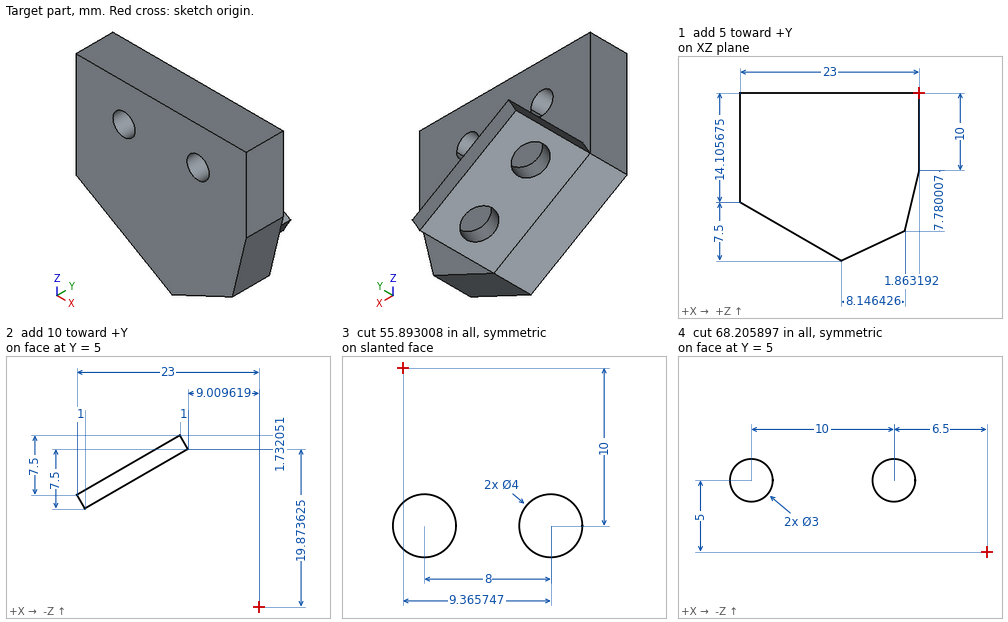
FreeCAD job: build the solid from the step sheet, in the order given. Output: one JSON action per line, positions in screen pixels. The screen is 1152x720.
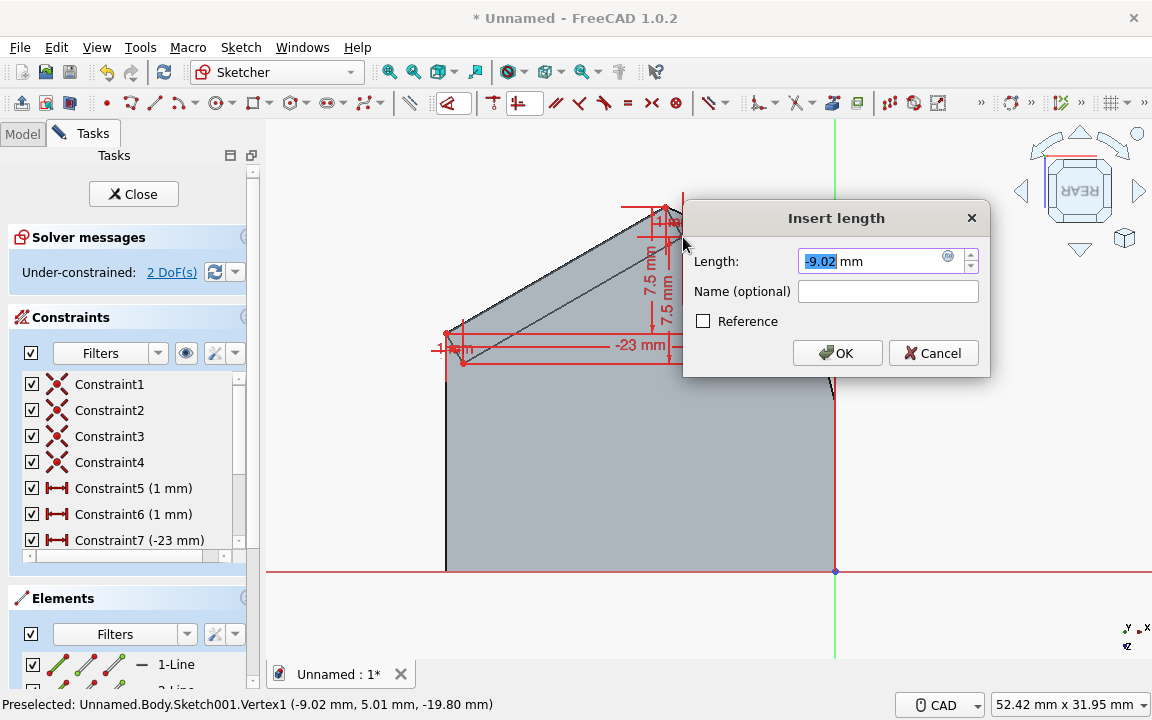
{"action": "type", "text": "-9.009619"}
{"action": "key", "text": "Return"}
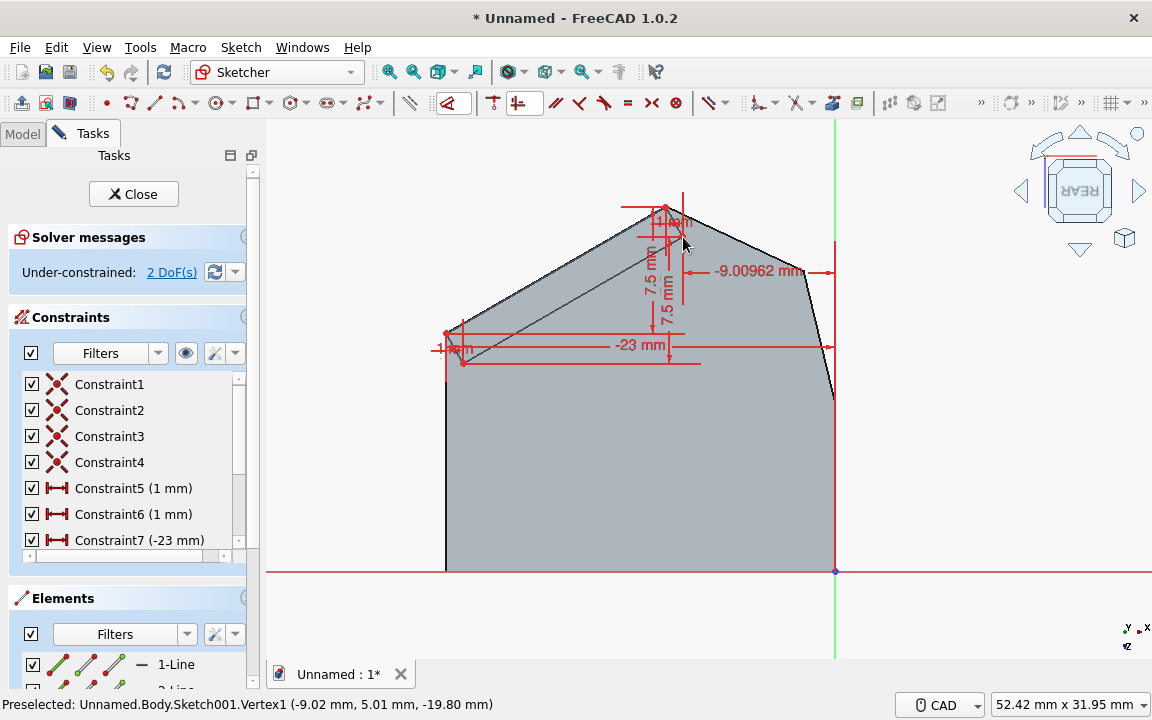
{"action": "scroll", "coordinate": [678, 228], "scroll_direction": "up", "scroll_amount": 2}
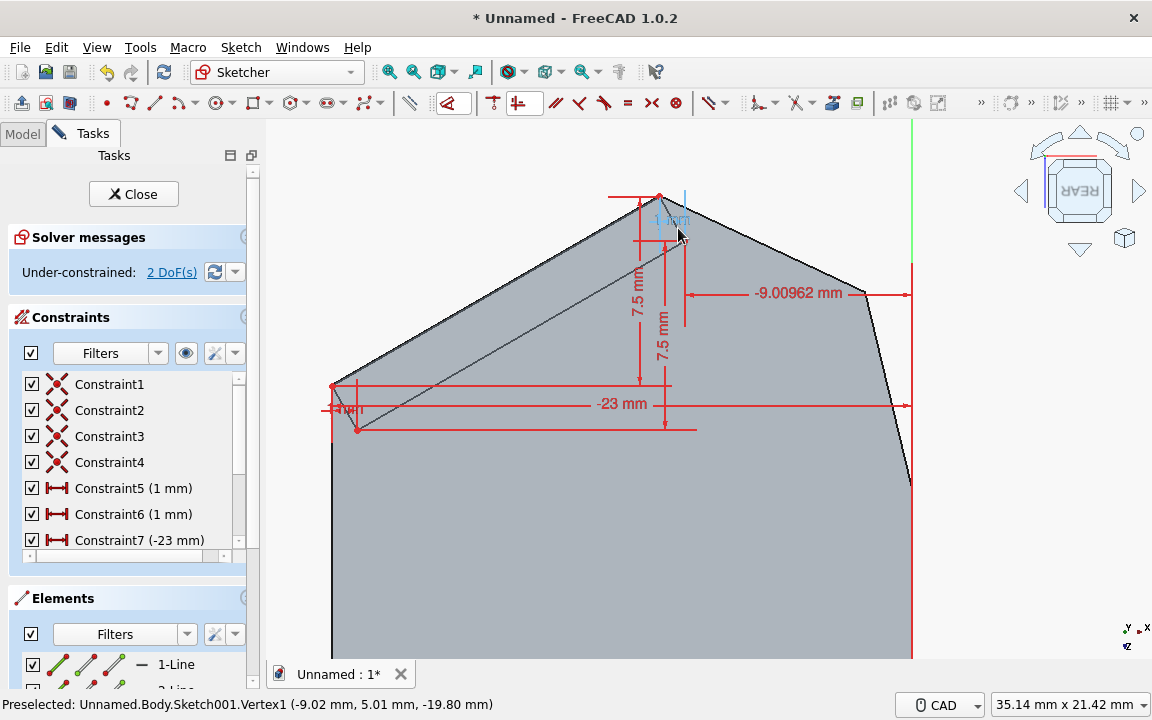
{"action": "left_click", "coordinate": [667, 210]}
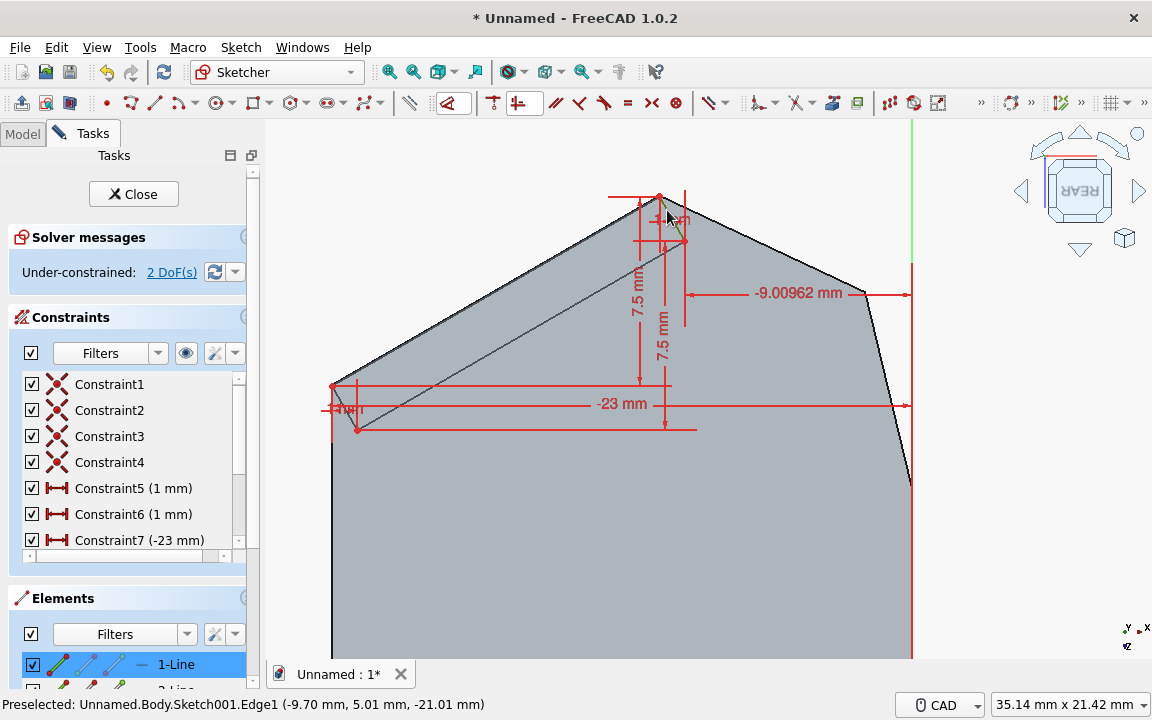
{"action": "key", "text": "i"}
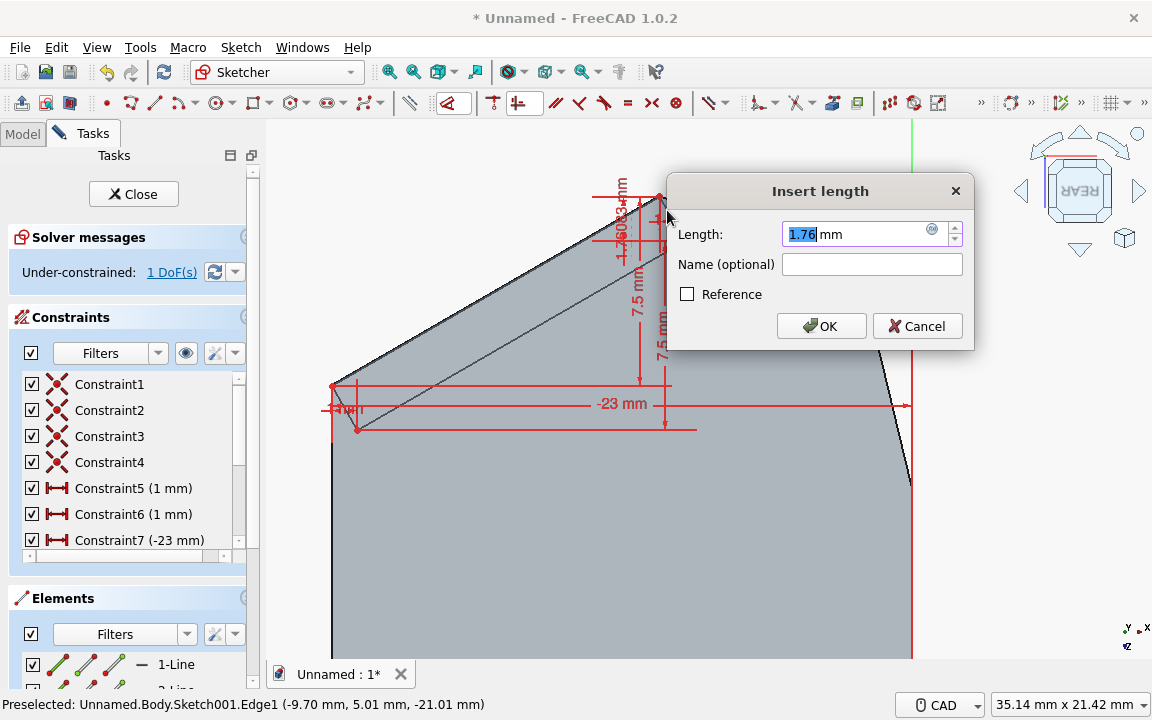
{"action": "type", "text": "1.732051"}
{"action": "key", "text": "Return"}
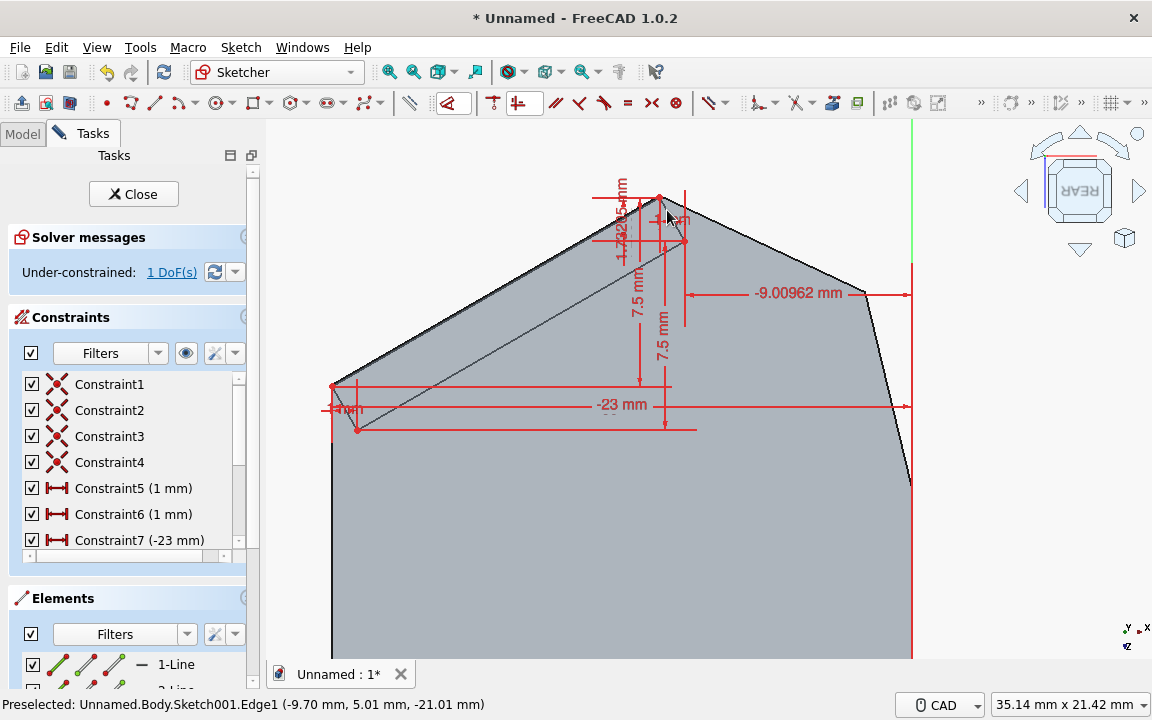
{"action": "left_click", "coordinate": [685, 241]}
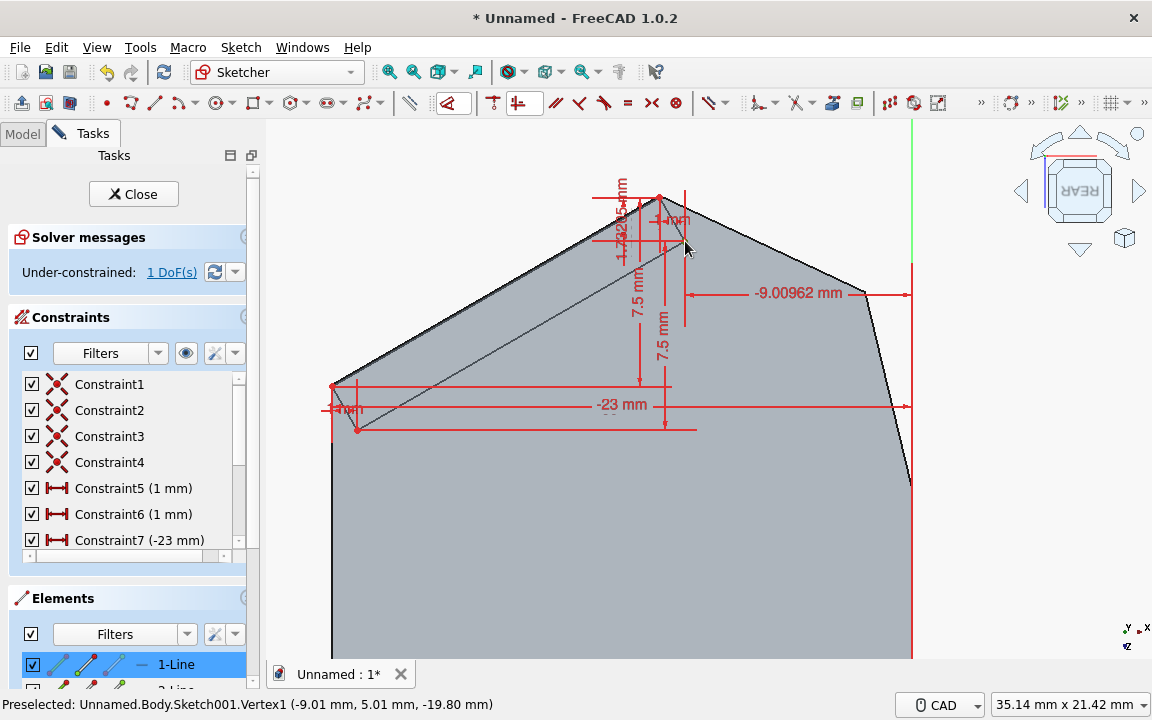
{"action": "key", "text": "i"}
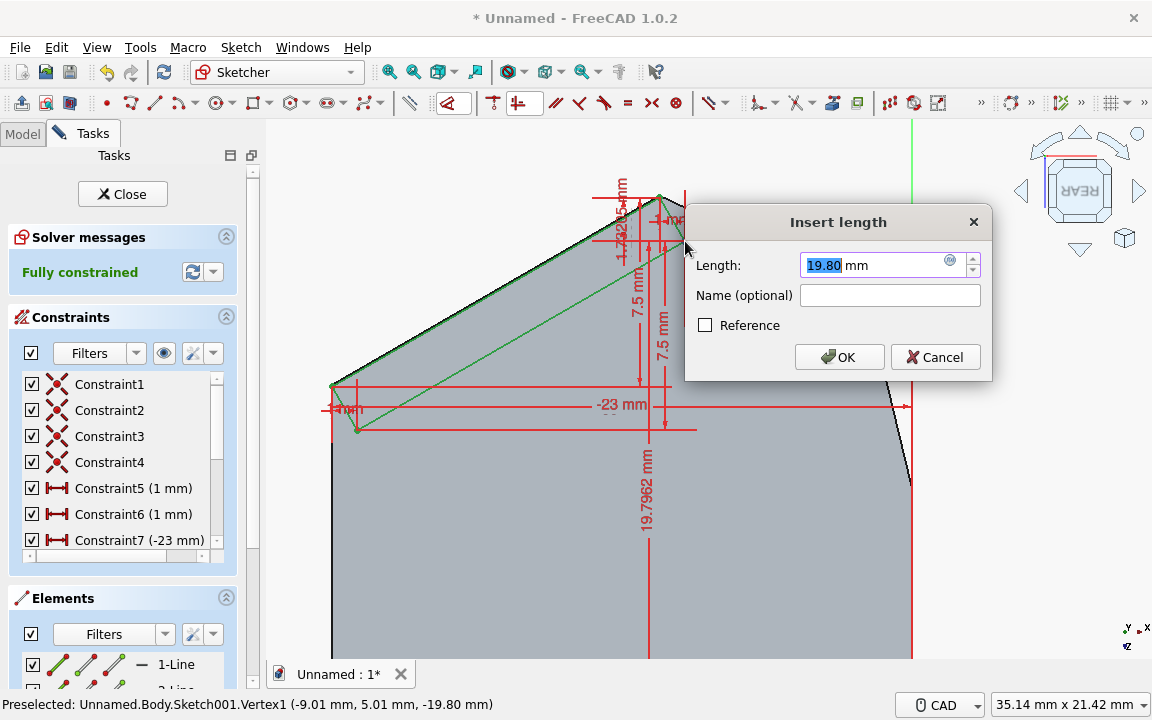
{"action": "type", "text": "19.873625"}
{"action": "key", "text": "Return"}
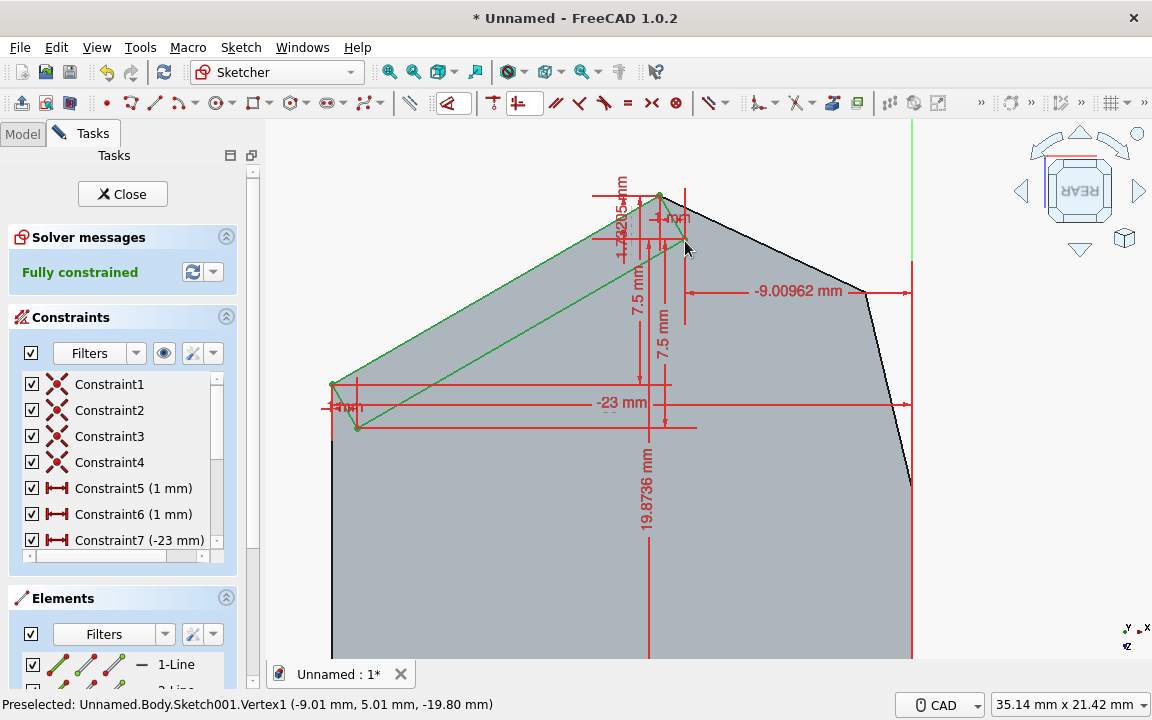
{"action": "left_click", "coordinate": [123, 194]}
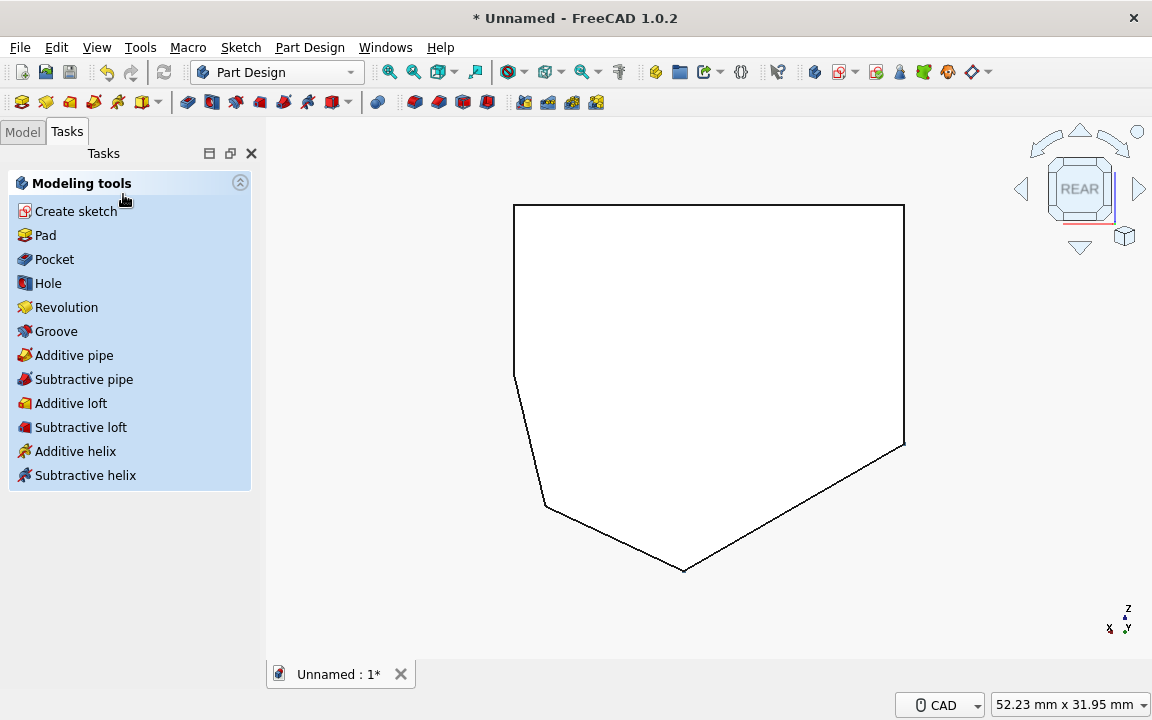
{"action": "left_click", "coordinate": [22, 102]}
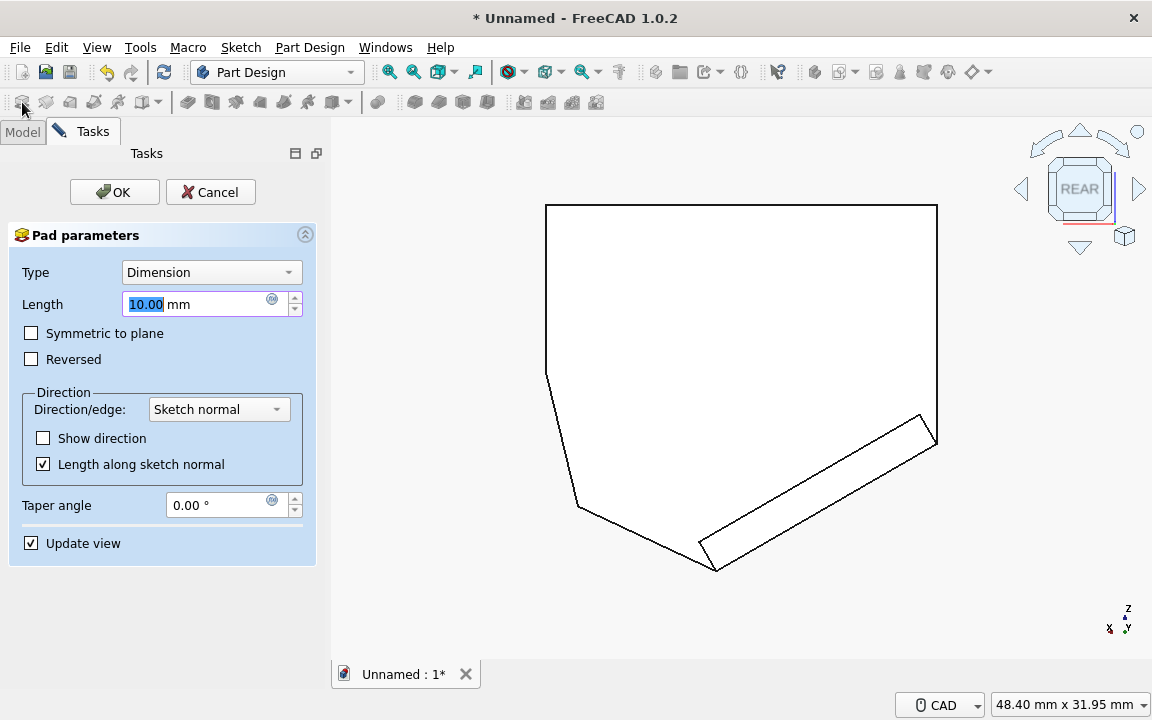
{"action": "type", "text": "10"}
{"action": "key", "text": "Tab"}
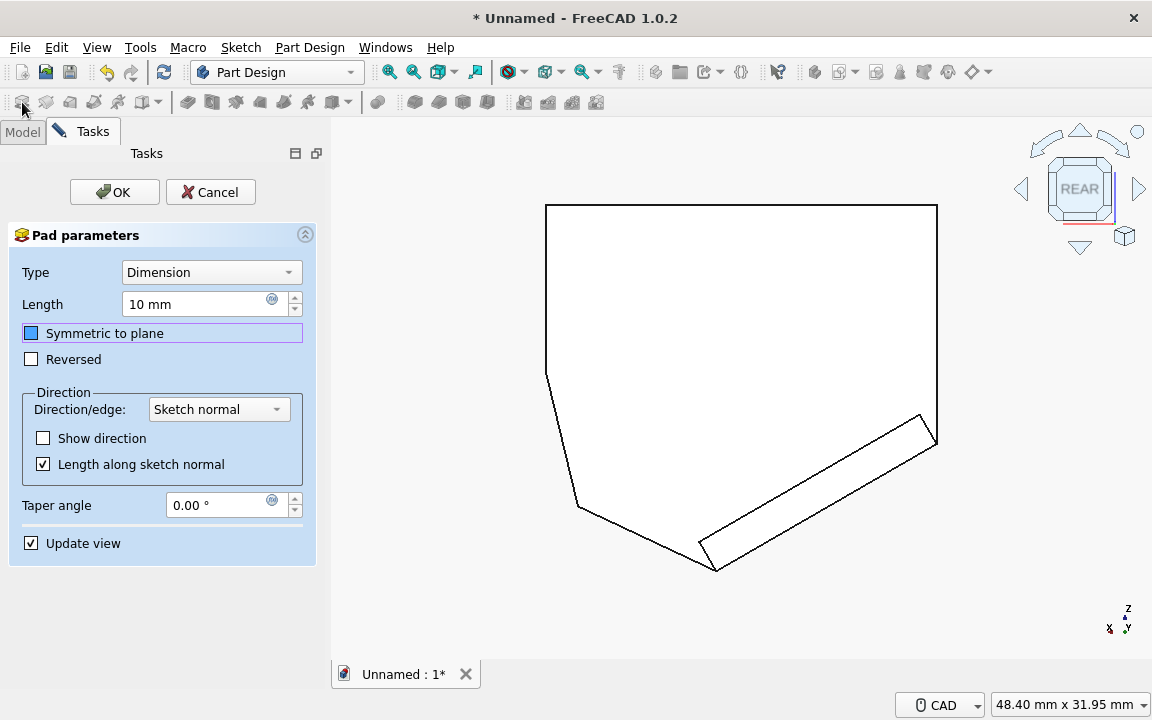
{"action": "left_click", "coordinate": [115, 192]}